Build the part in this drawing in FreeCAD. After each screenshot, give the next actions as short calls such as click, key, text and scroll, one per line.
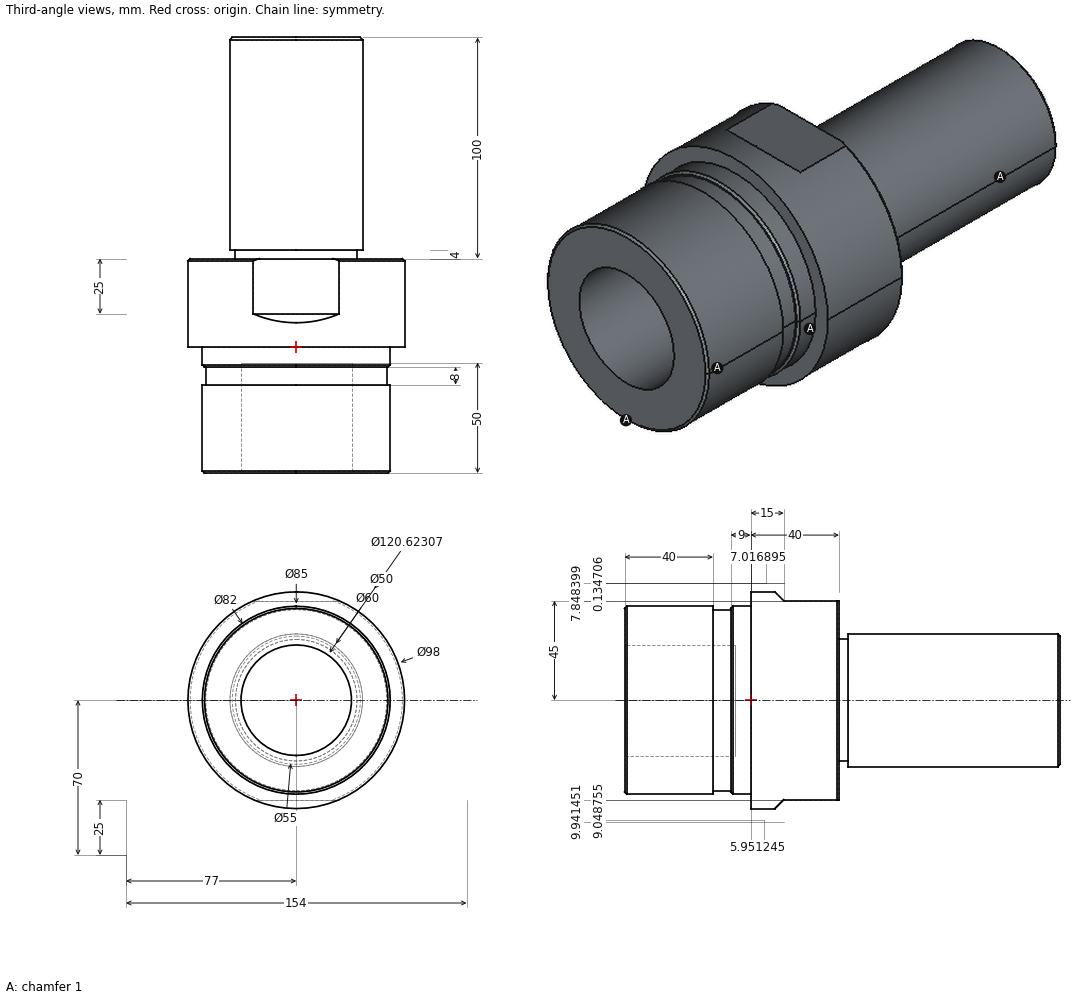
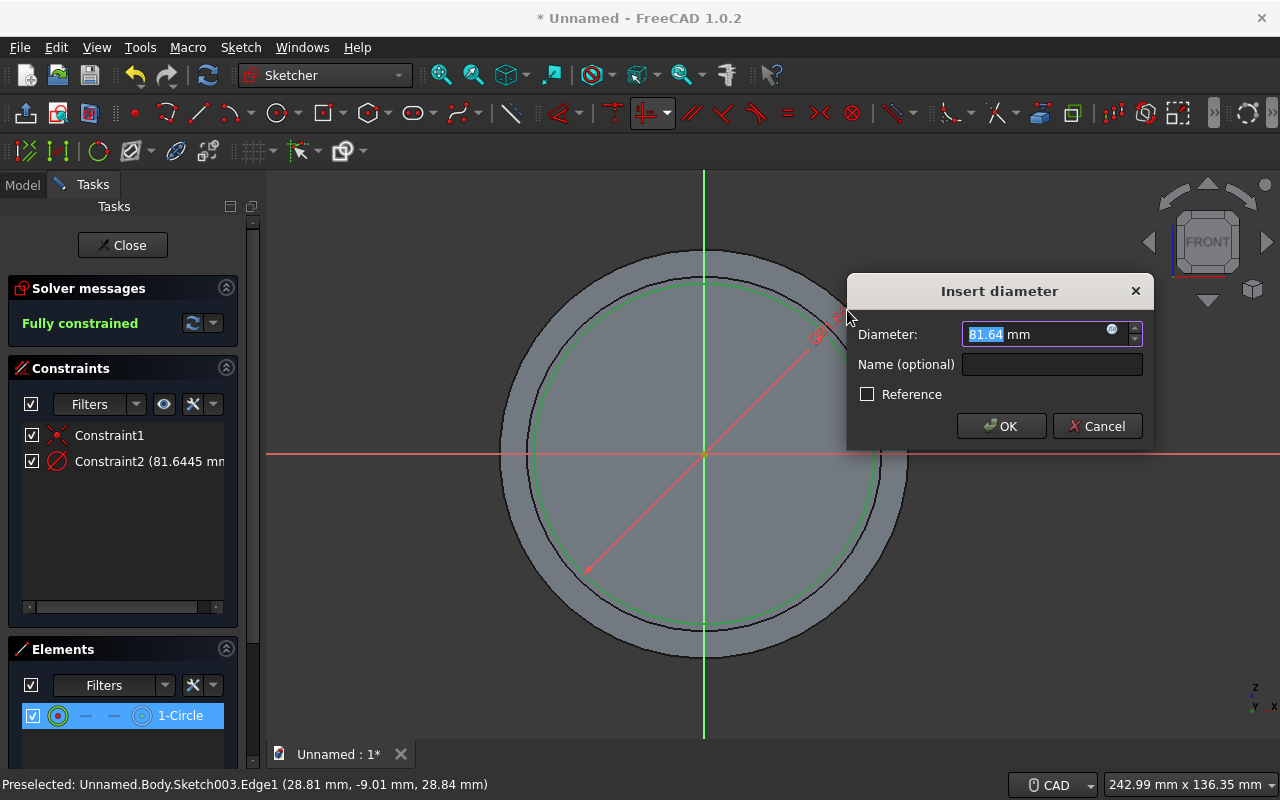
text(82)
key(Return)
key(Escape)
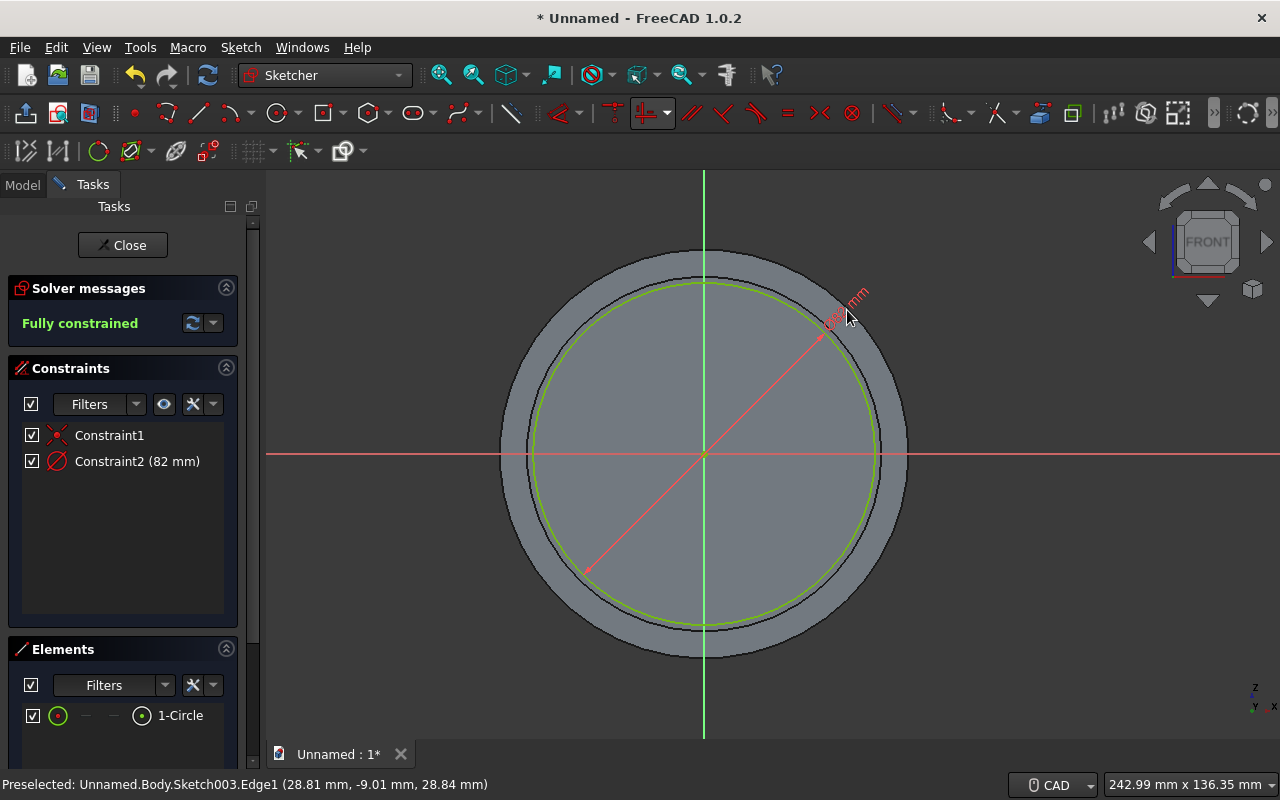
click(123, 245)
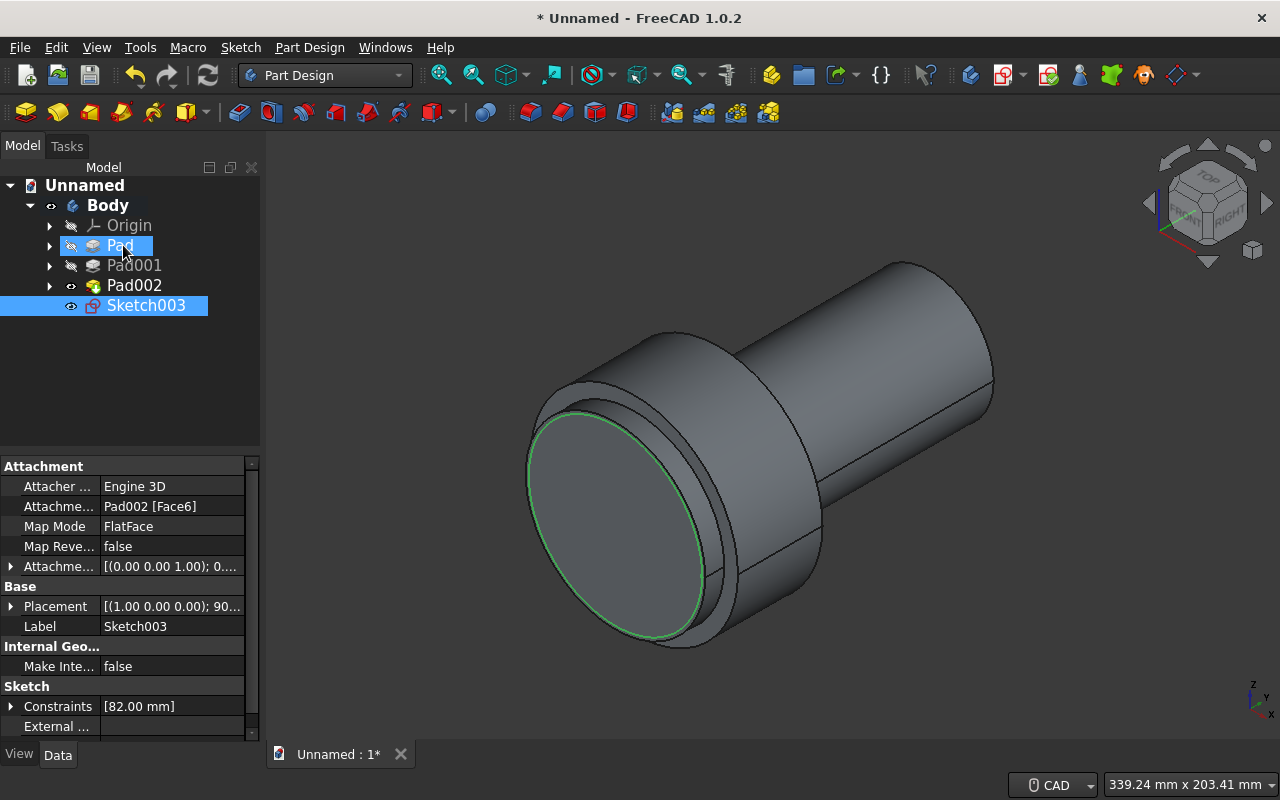
click(26, 112)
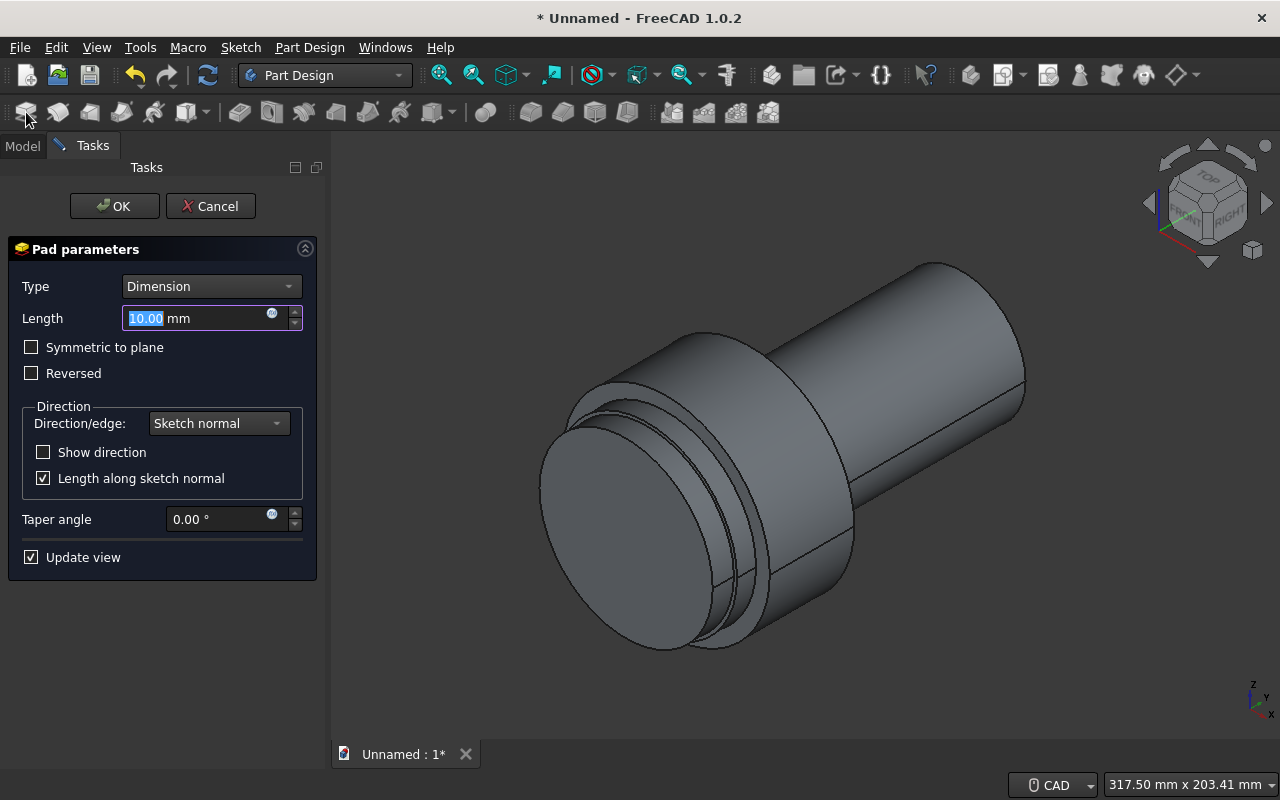
text(8)
key(Tab)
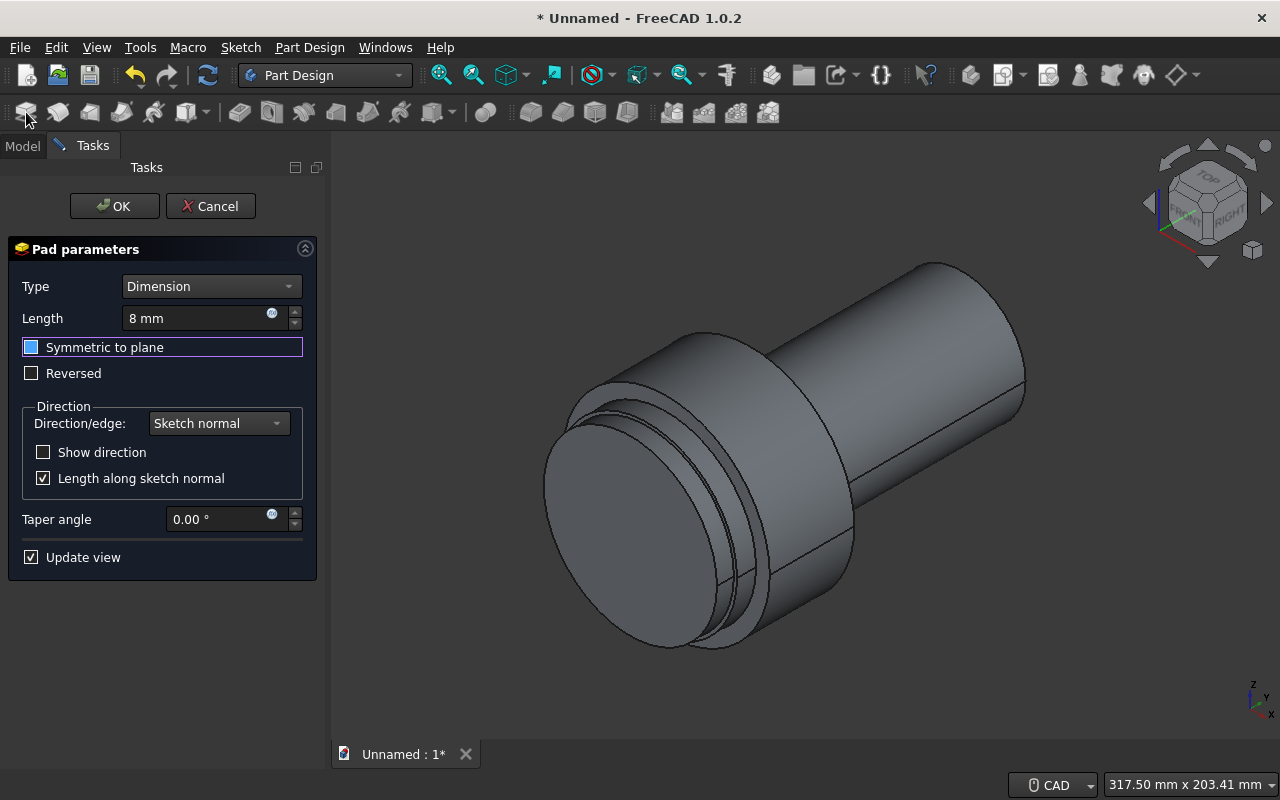
click(115, 206)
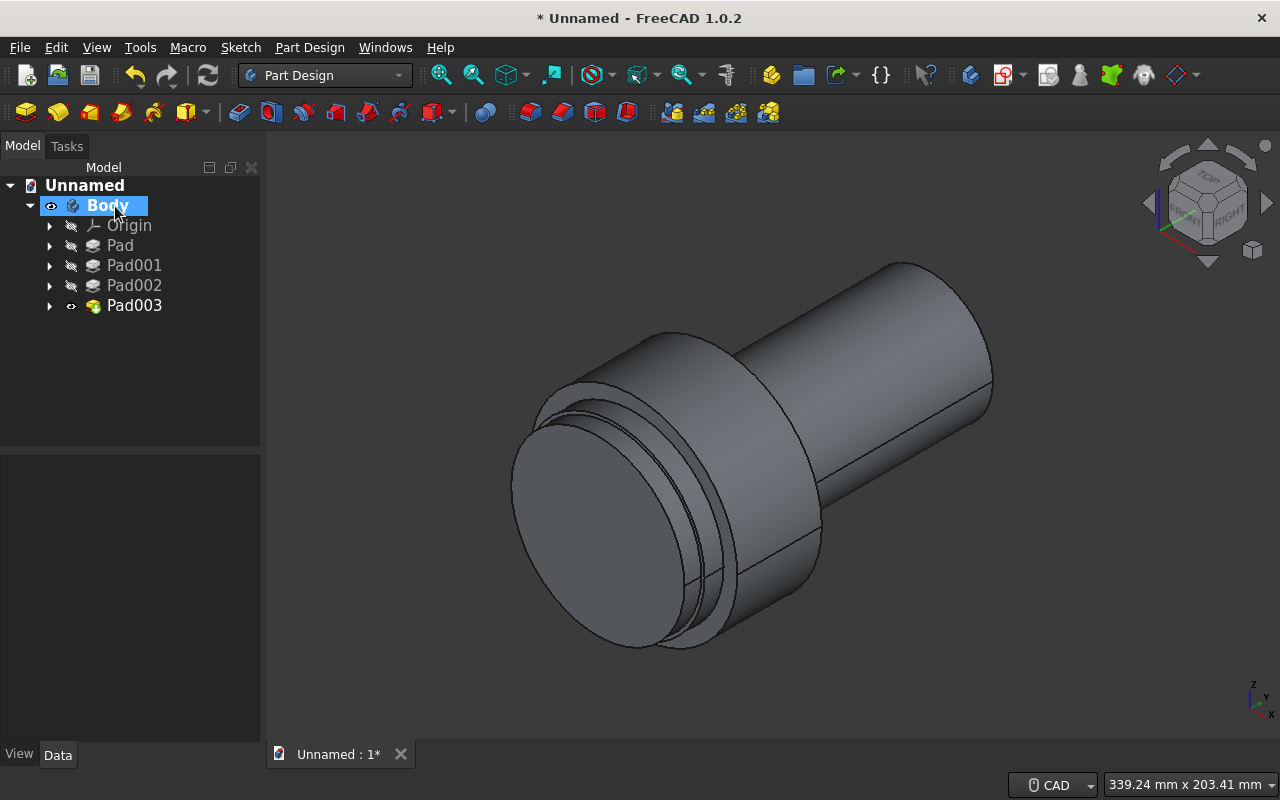
click(598, 535)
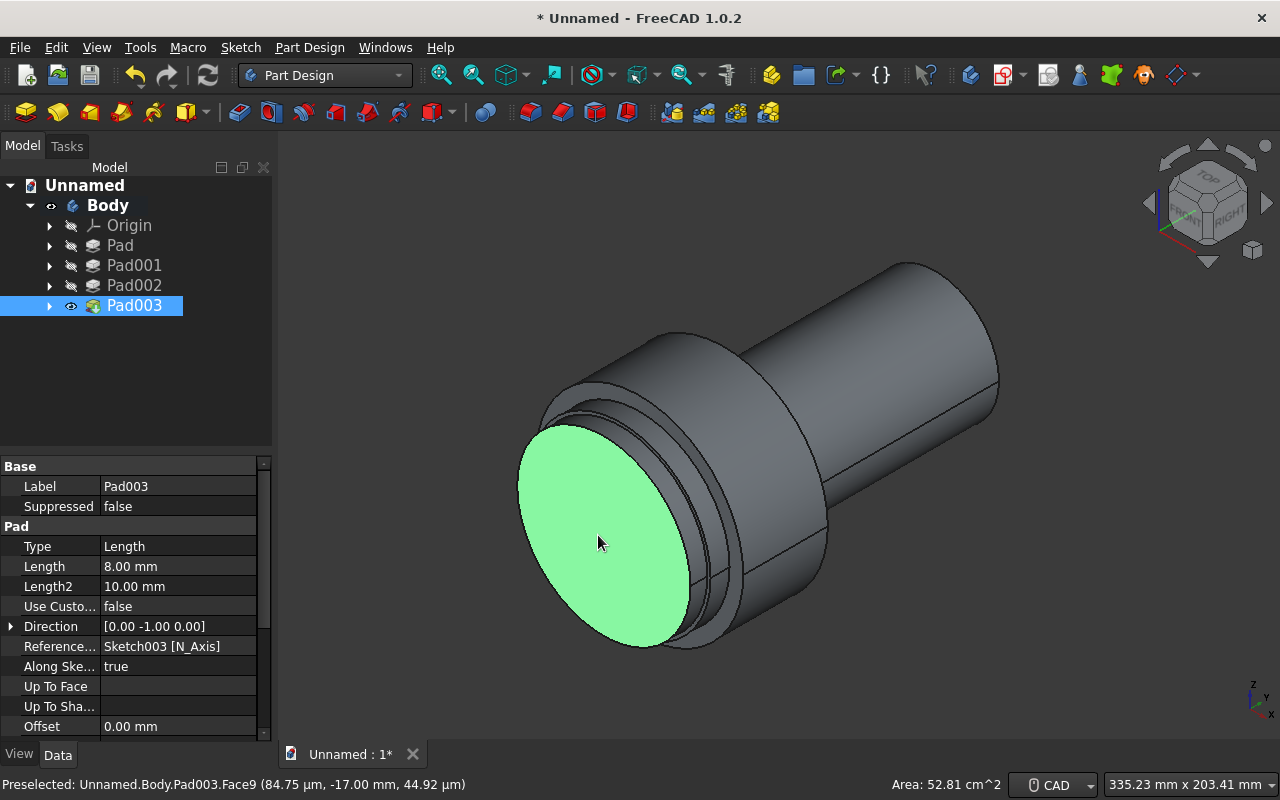
click(1004, 76)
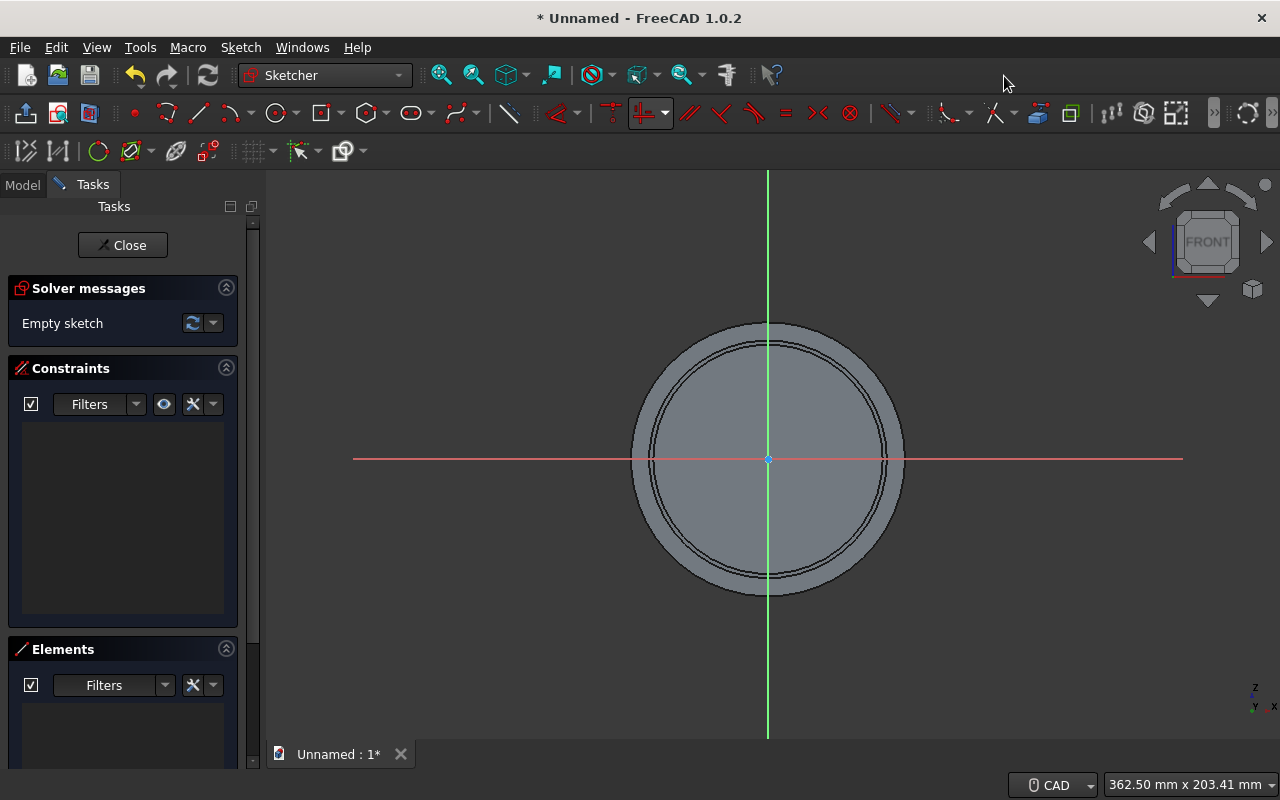
scroll(897, 469, up, 2)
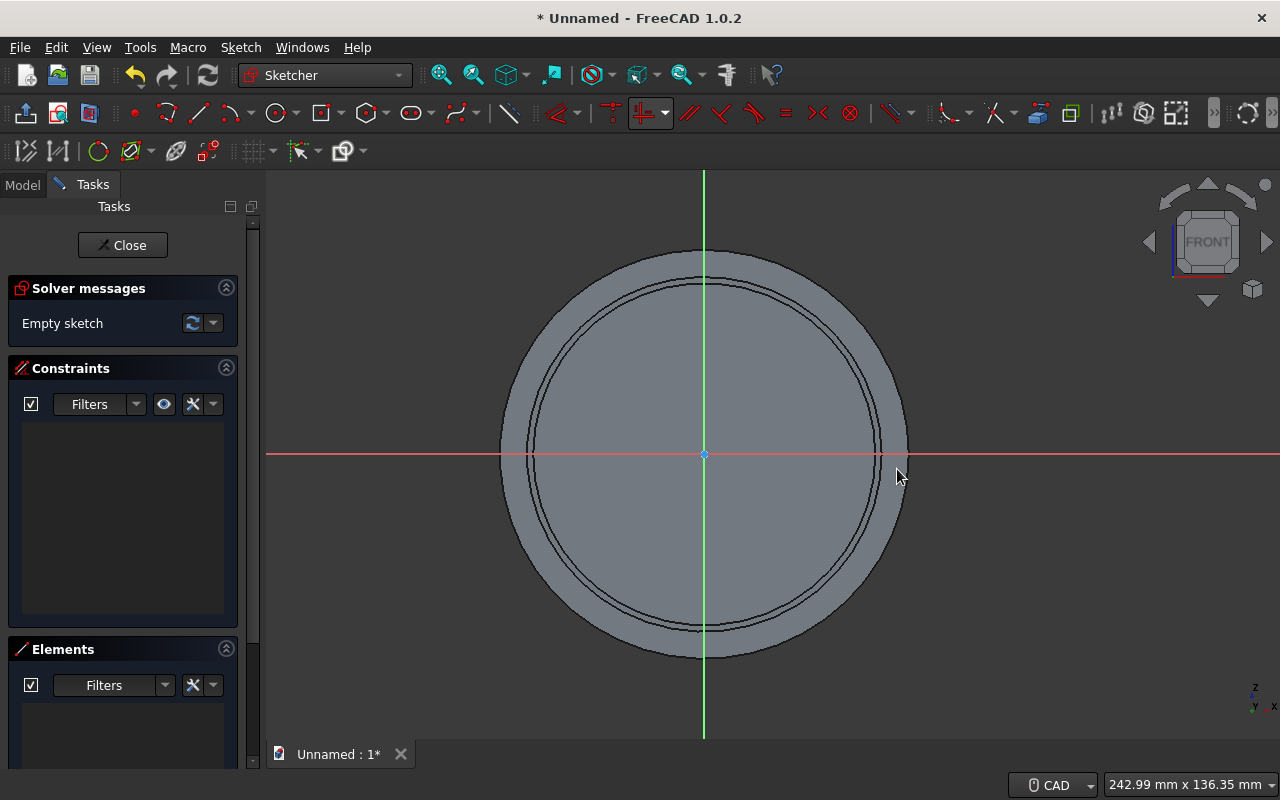
click(276, 114)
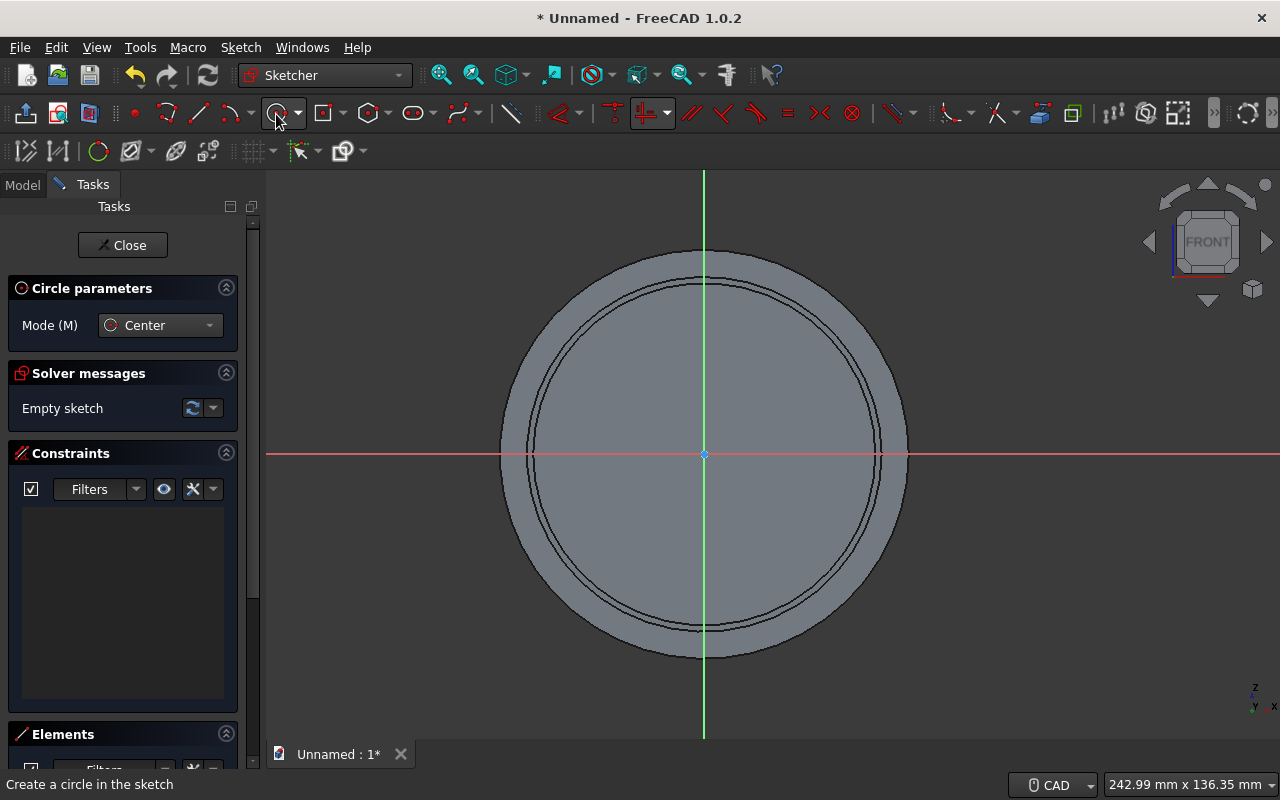
click(704, 454)
click(830, 329)
key(Escape)